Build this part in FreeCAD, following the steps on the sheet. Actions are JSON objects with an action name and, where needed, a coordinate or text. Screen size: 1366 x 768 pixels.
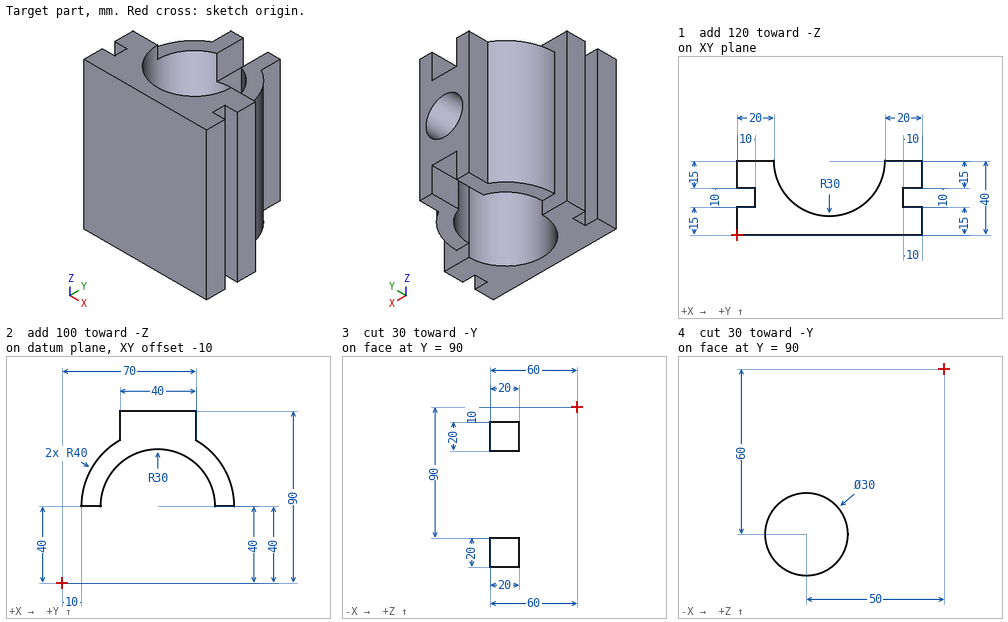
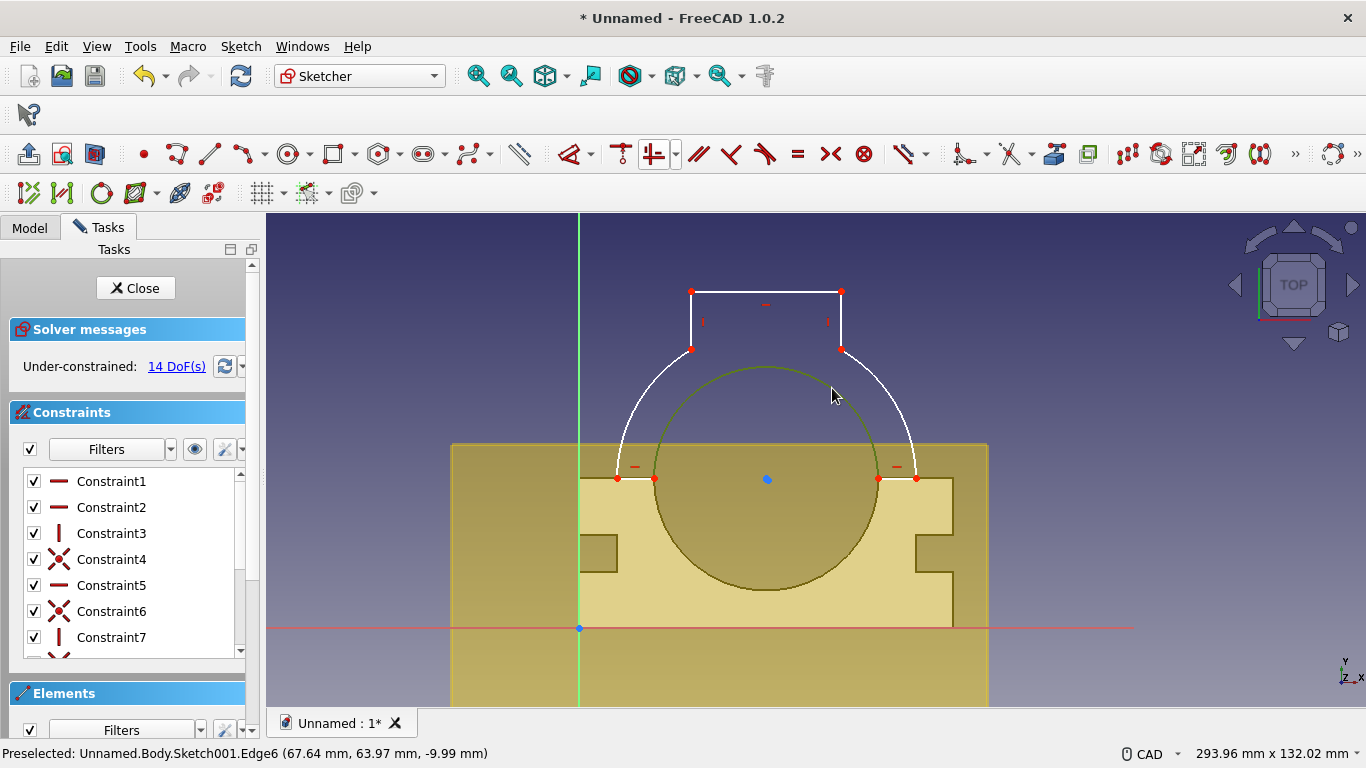
{"action": "left_click", "coordinate": [908, 433]}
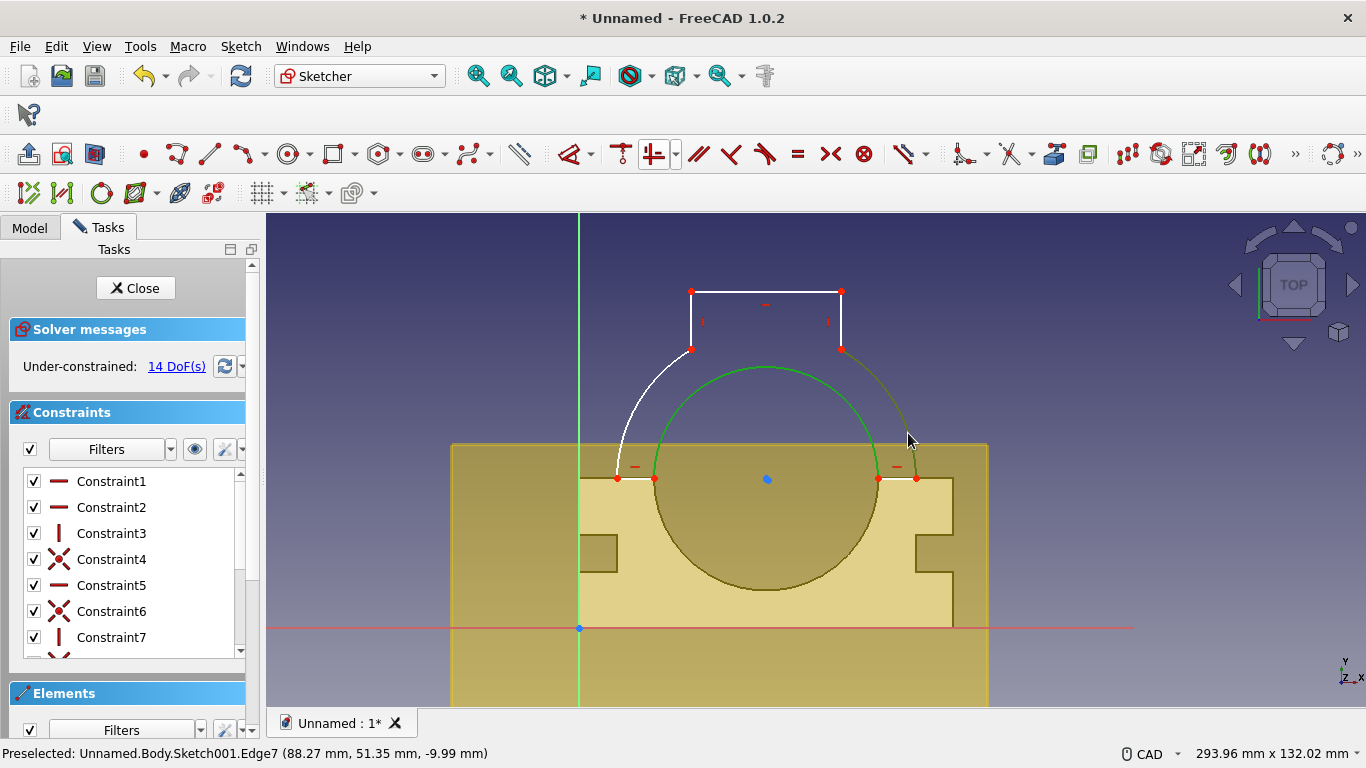
{"action": "left_click", "coordinate": [621, 154]}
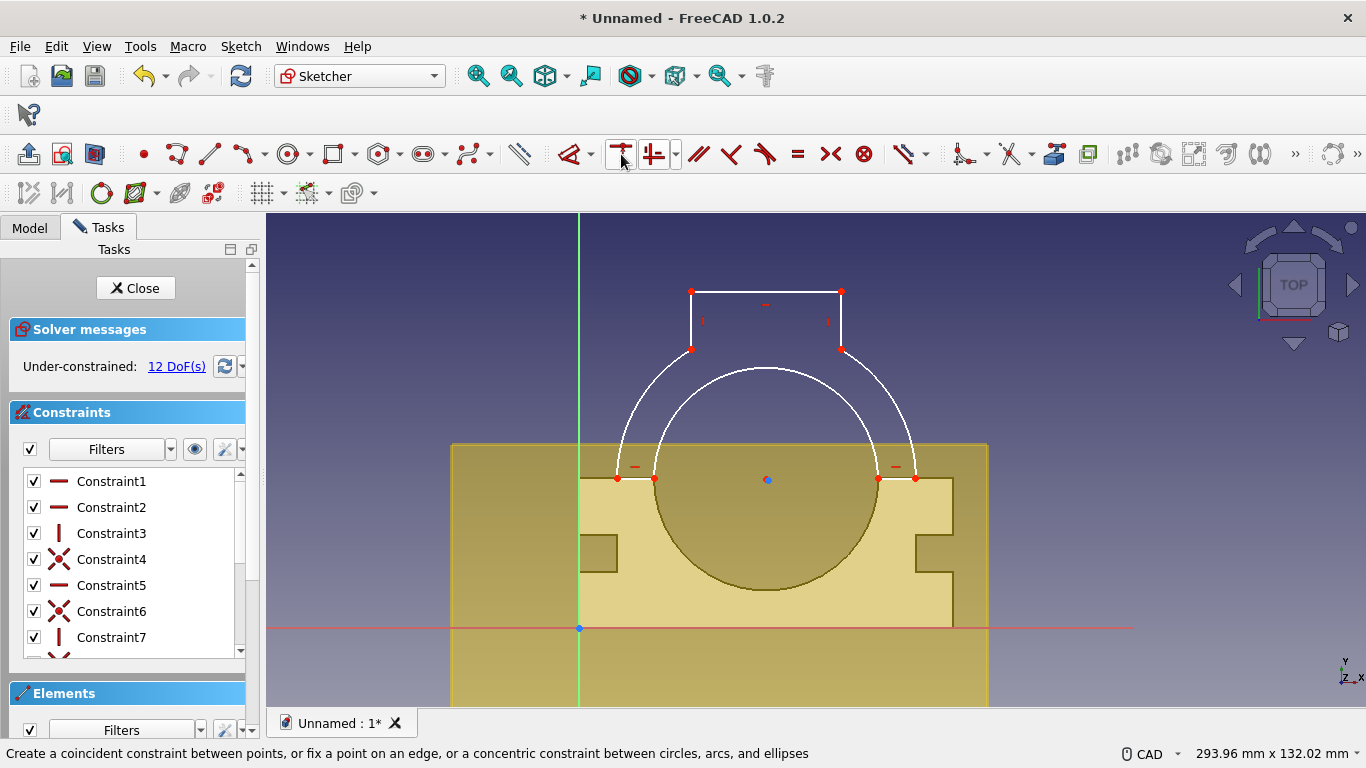
{"action": "left_click", "coordinate": [832, 389]}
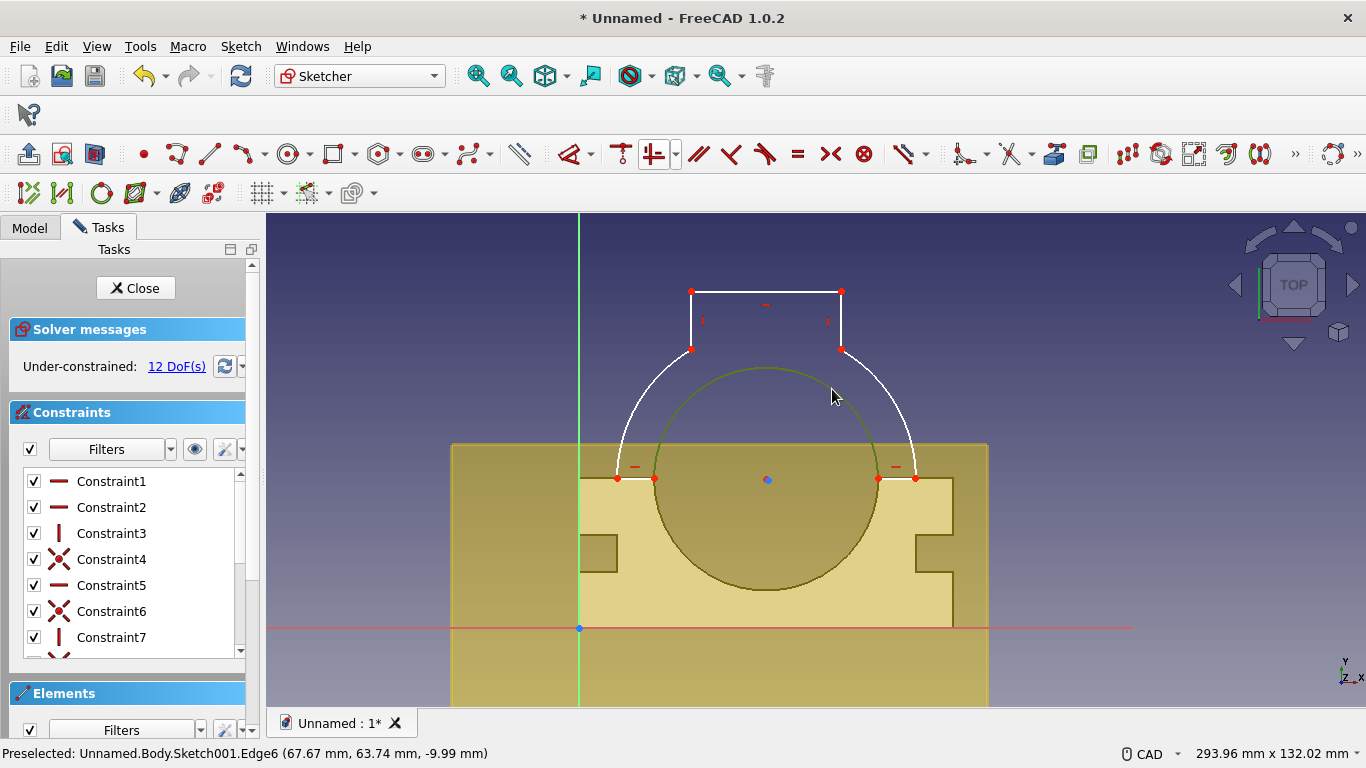
{"action": "left_click", "coordinate": [655, 380]}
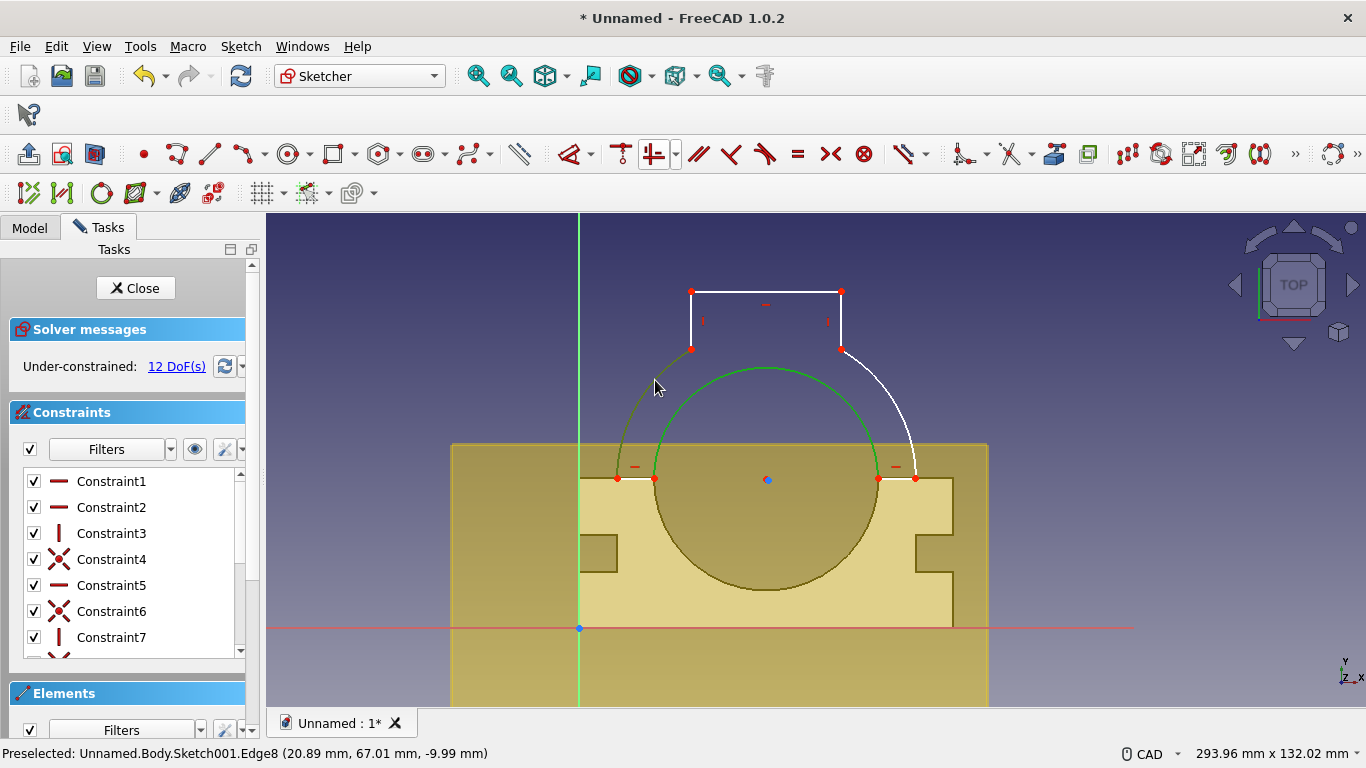
{"action": "left_click", "coordinate": [621, 154]}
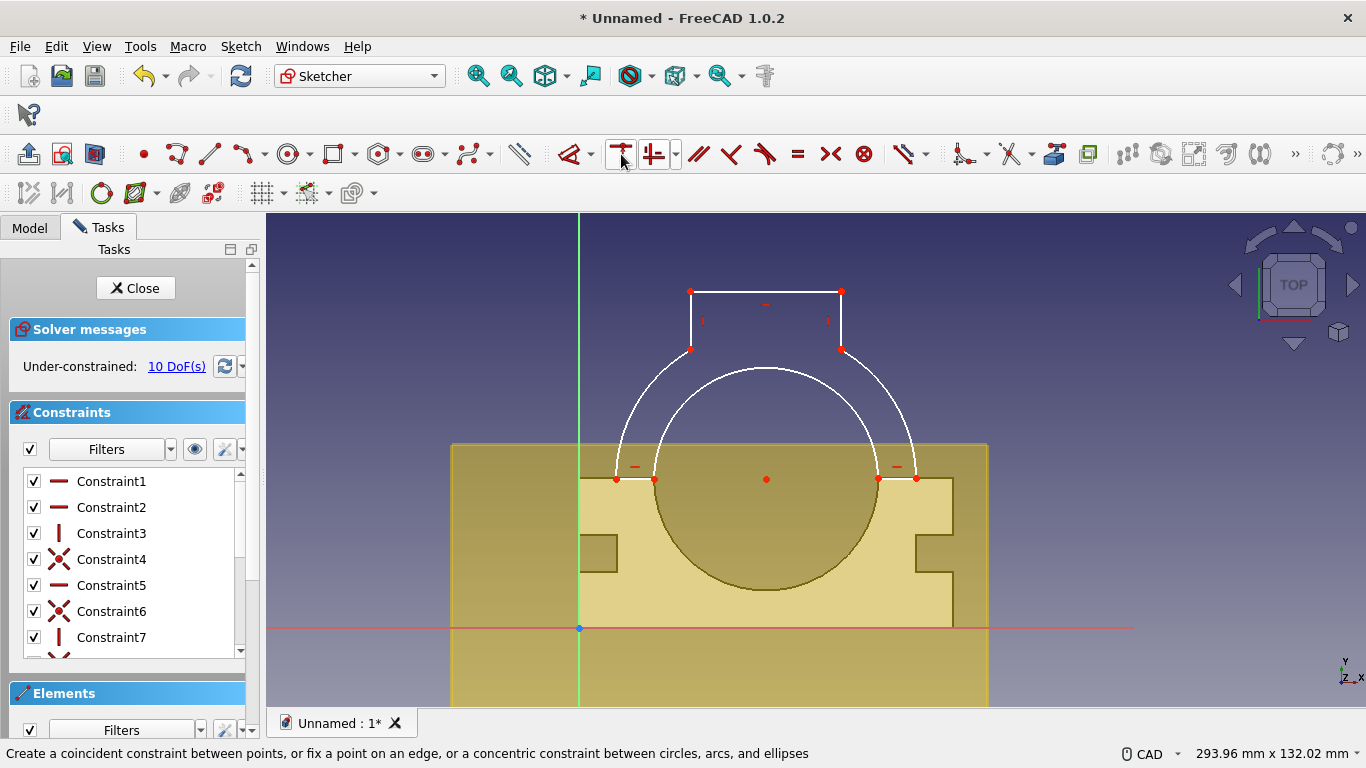
{"action": "left_click", "coordinate": [909, 433]}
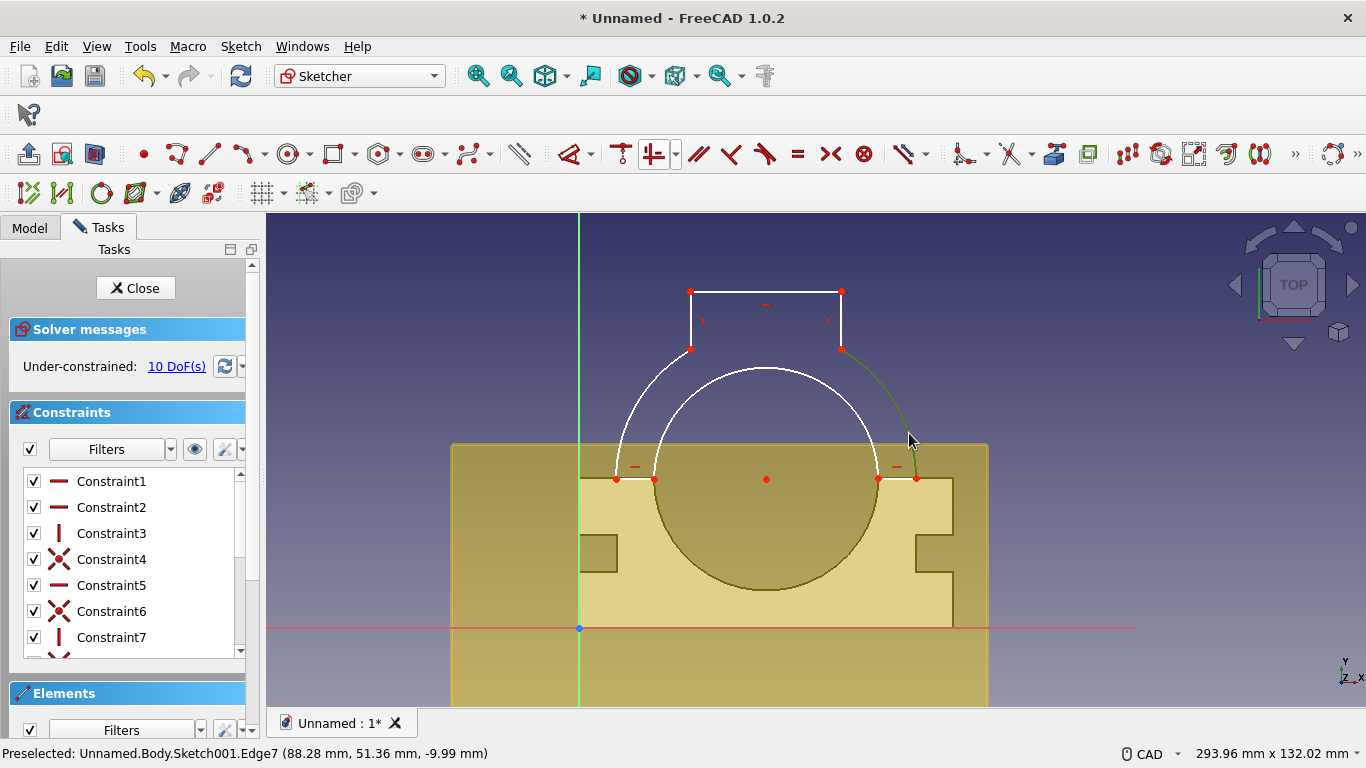
{"action": "left_click", "coordinate": [655, 379]}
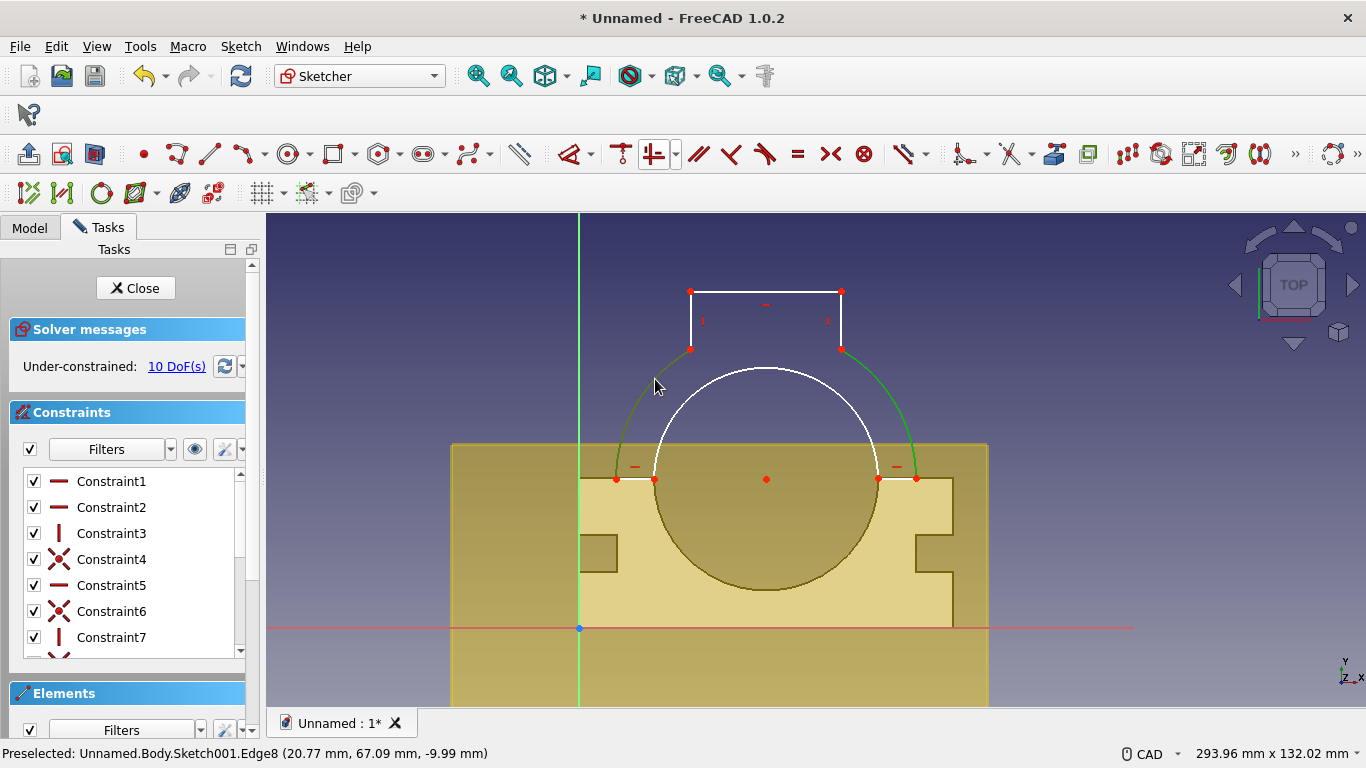
{"action": "left_click", "coordinate": [798, 154]}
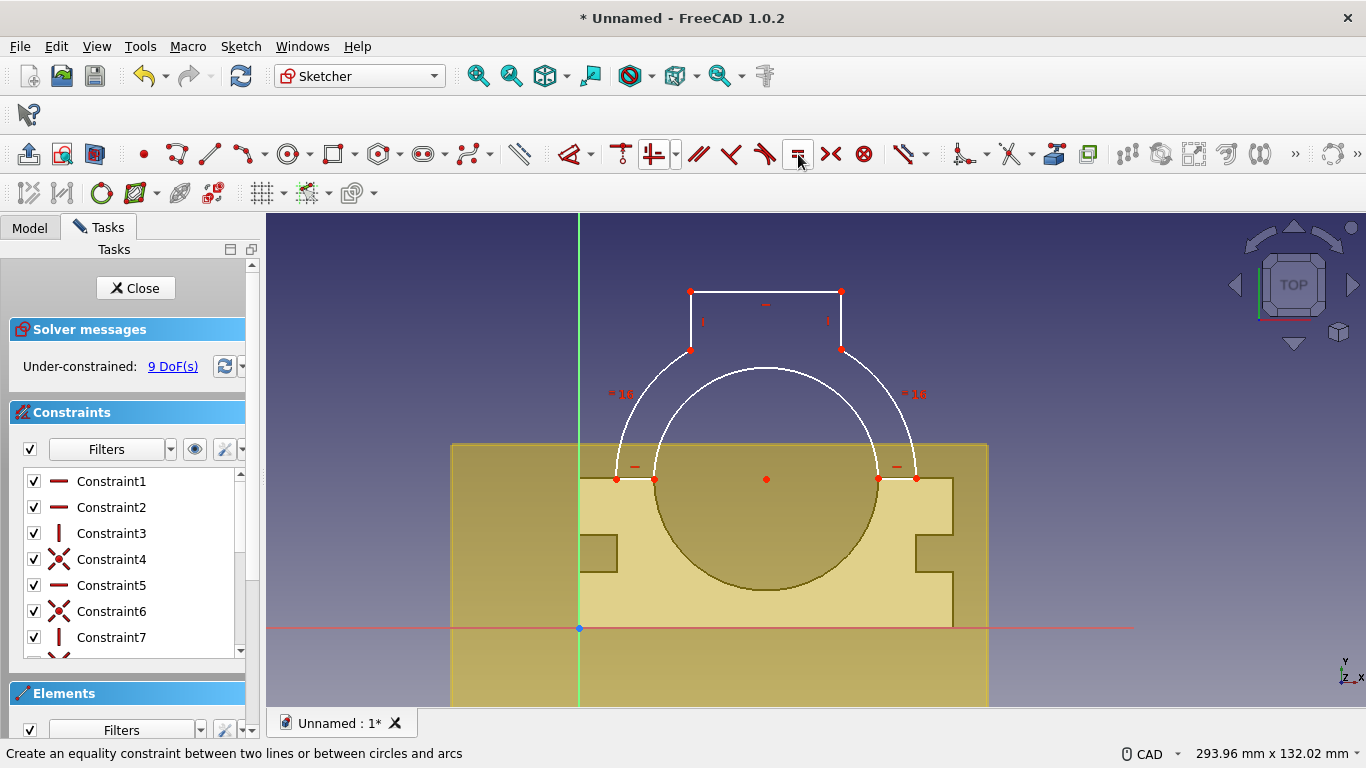
{"action": "left_click", "coordinate": [568, 154]}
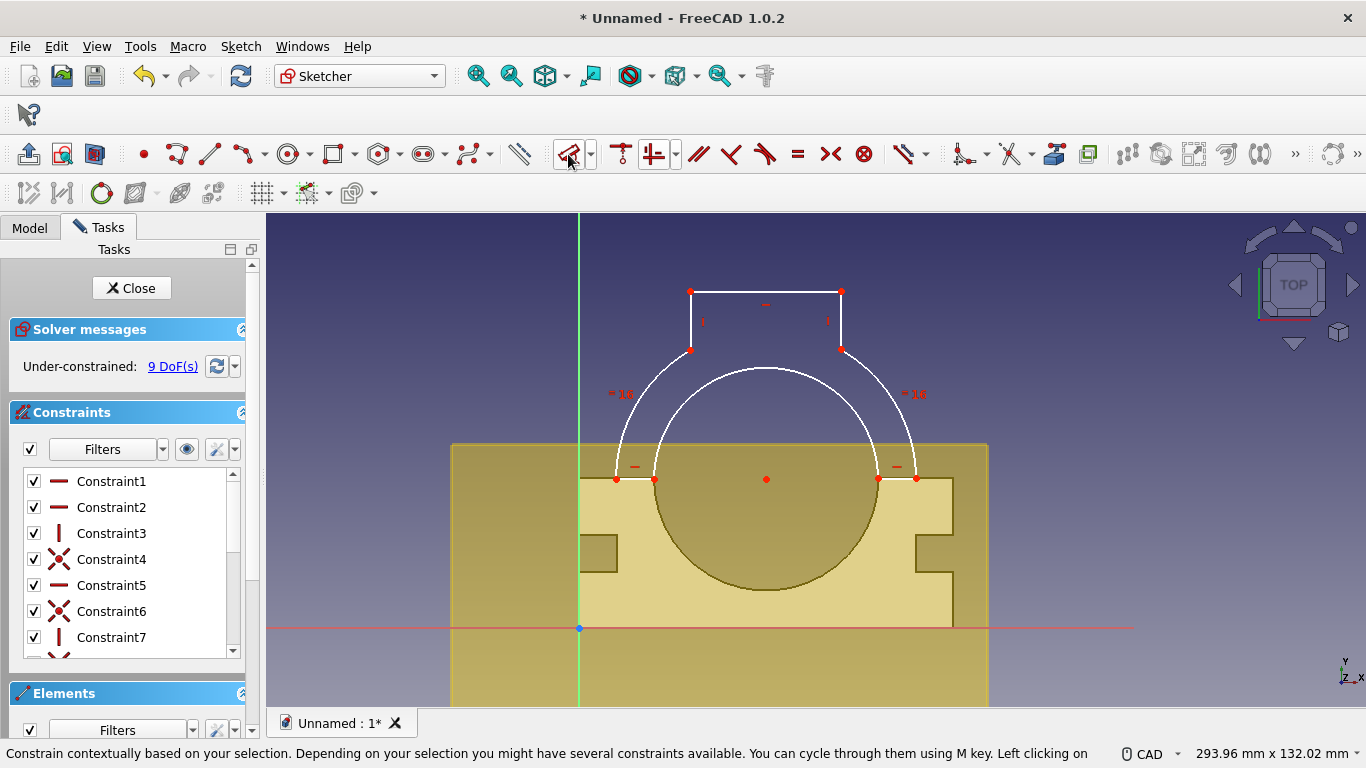
{"action": "left_click", "coordinate": [832, 389]}
{"action": "left_click", "coordinate": [784, 337]}